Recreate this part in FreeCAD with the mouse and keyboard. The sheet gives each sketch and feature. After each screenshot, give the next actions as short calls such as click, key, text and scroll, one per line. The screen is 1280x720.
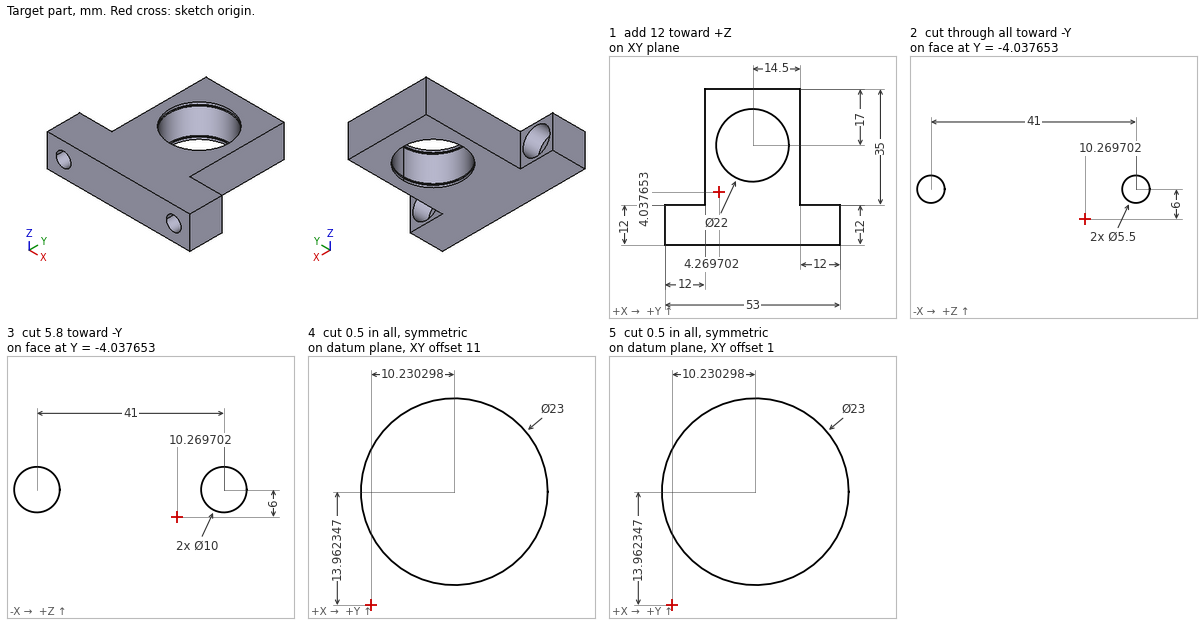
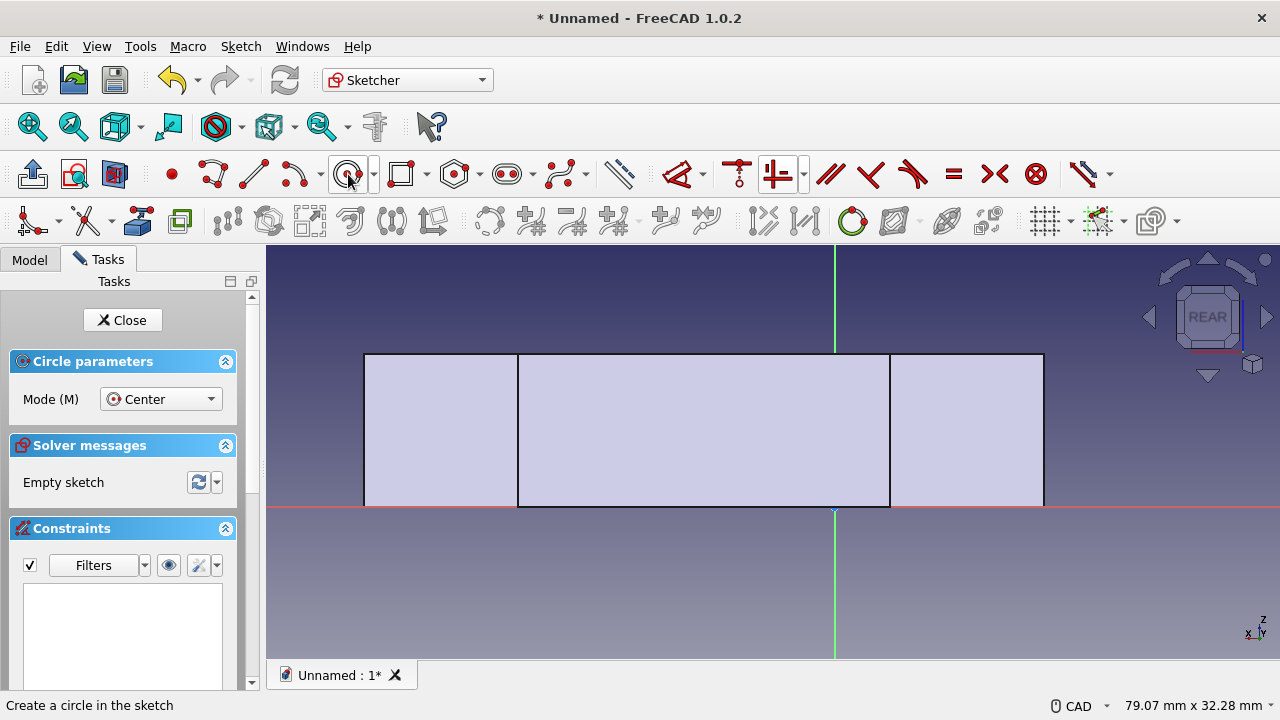
click(967, 431)
click(992, 406)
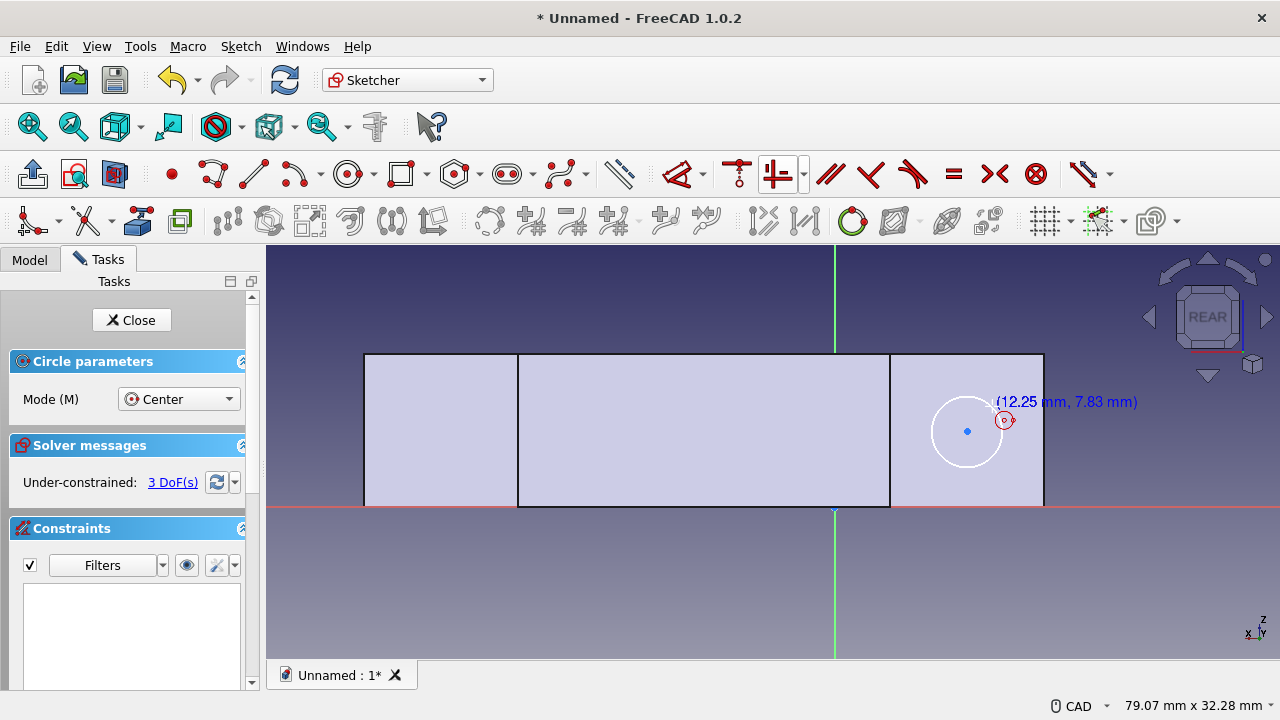
click(441, 431)
click(466, 406)
key(Escape)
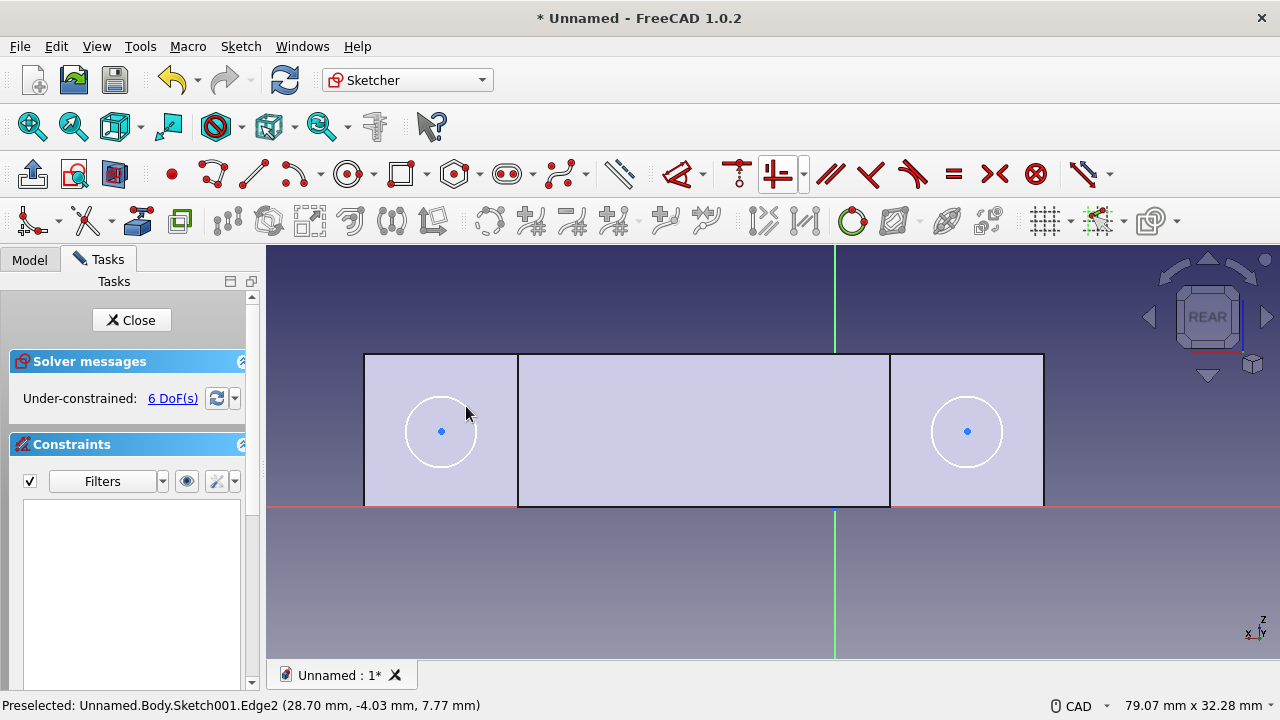
click(992, 407)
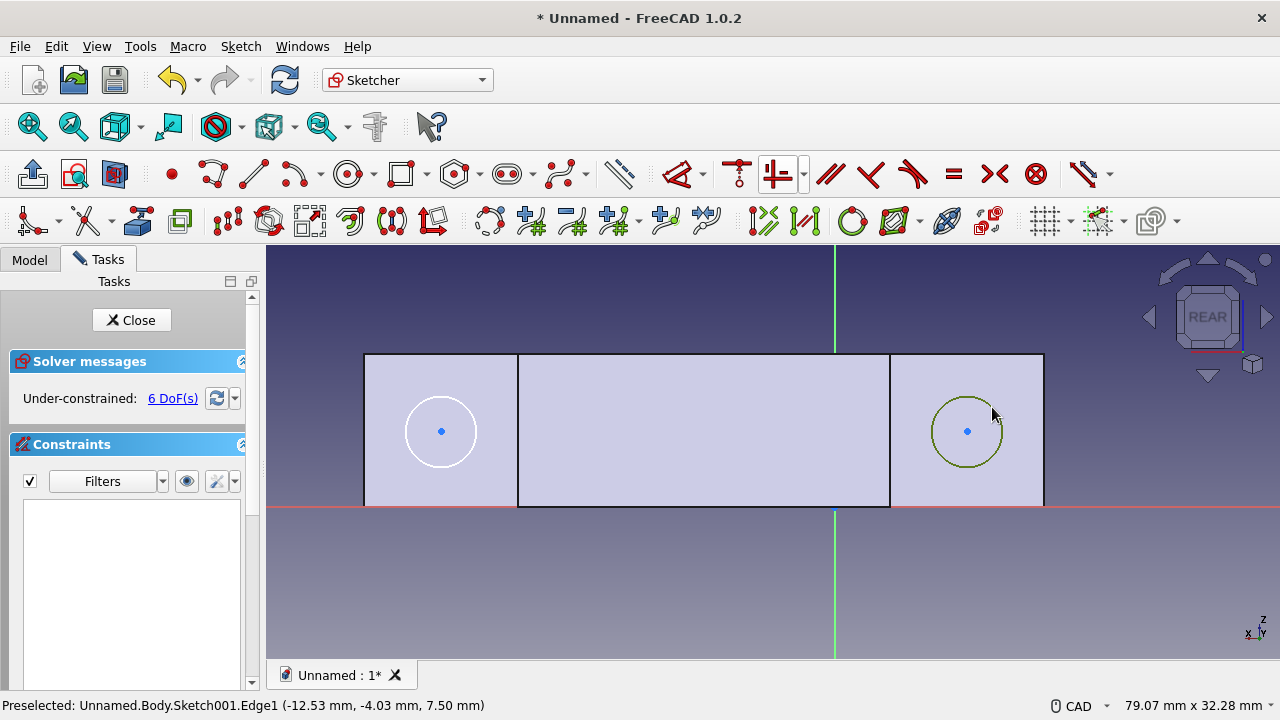
click(466, 407)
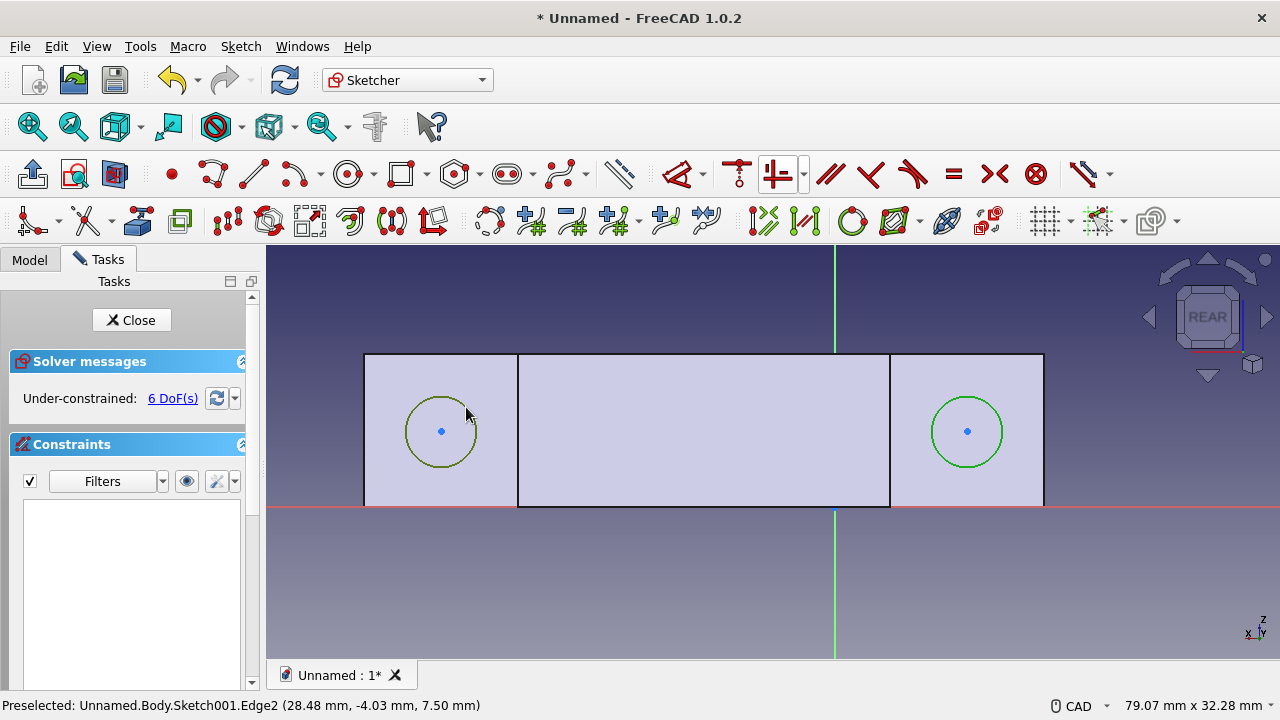
click(954, 174)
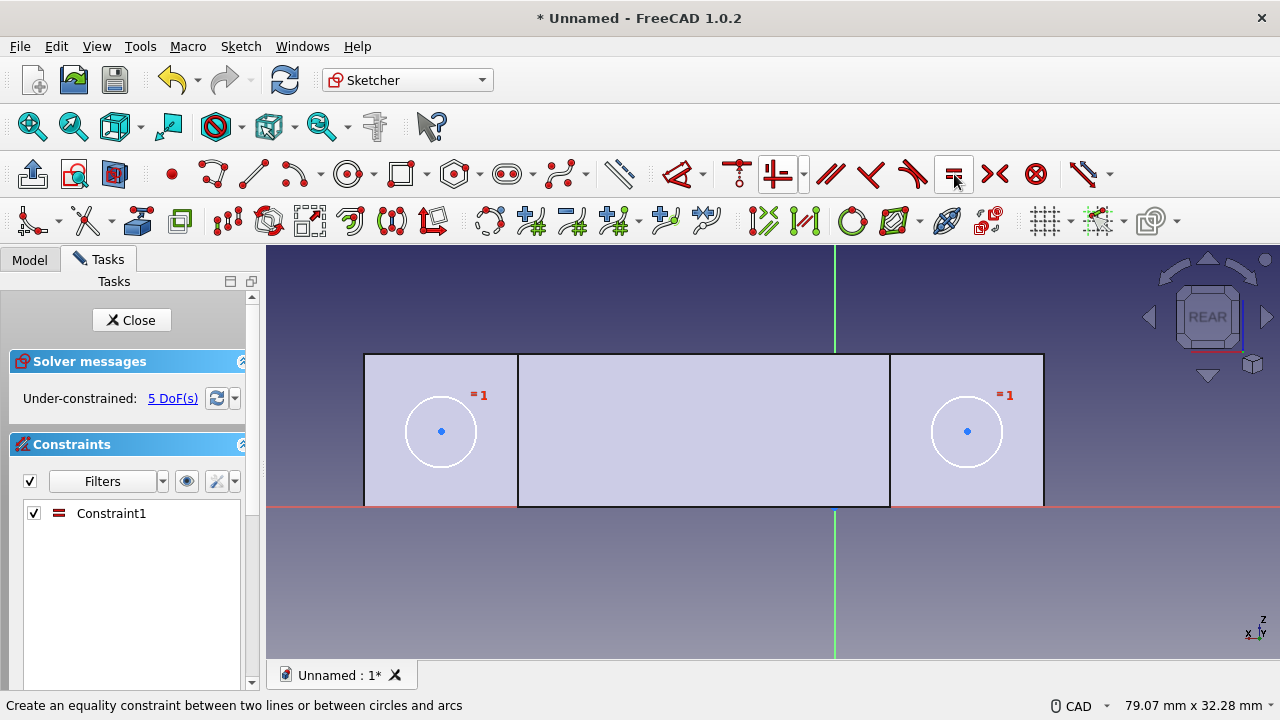
click(967, 432)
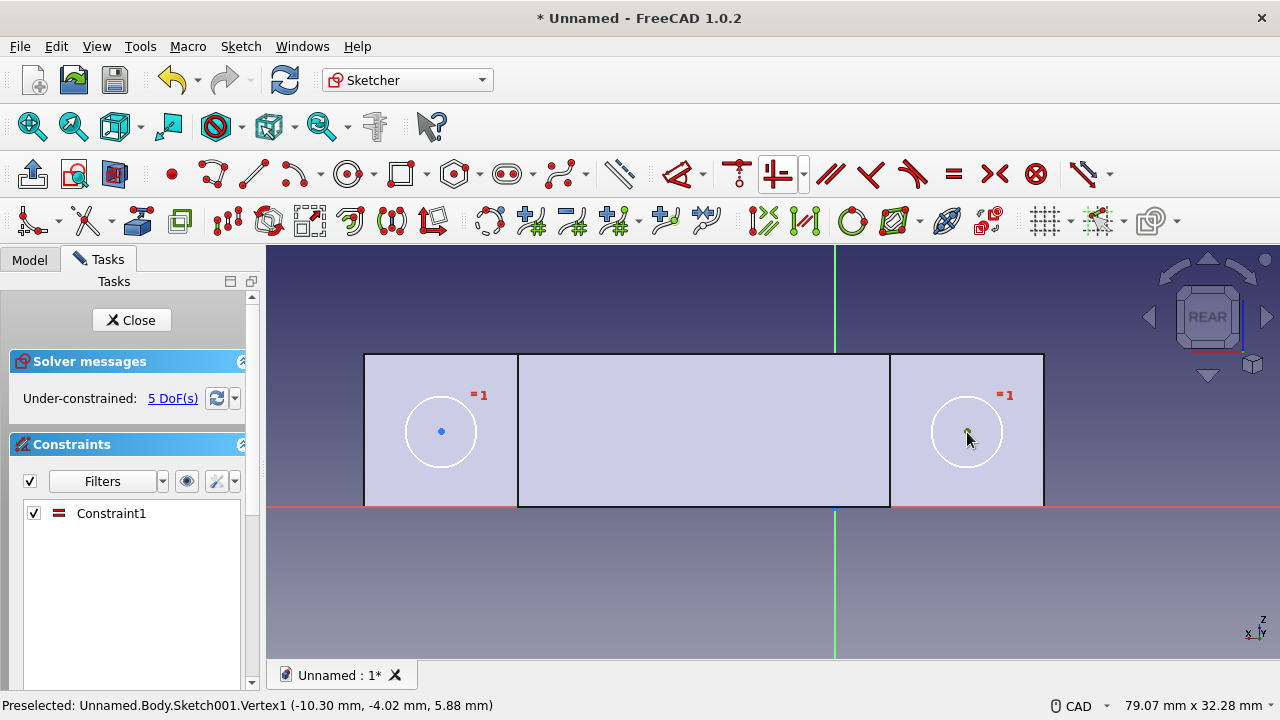
click(441, 432)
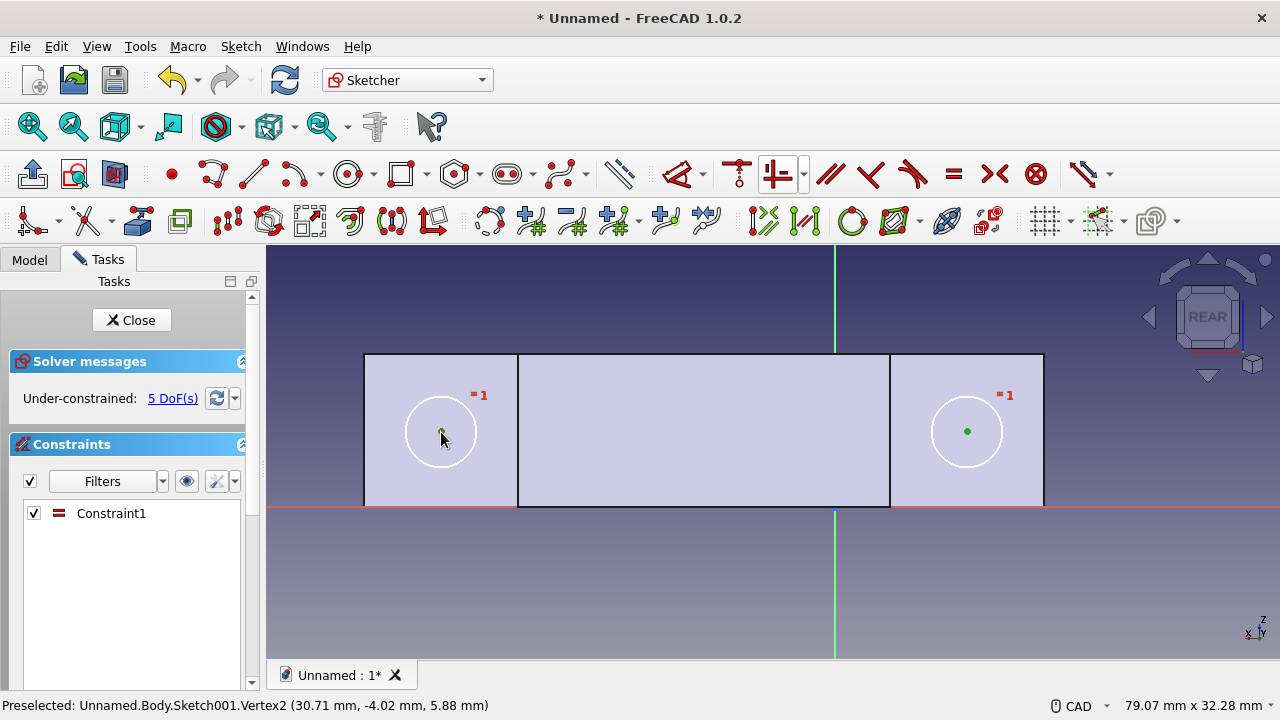
key(h)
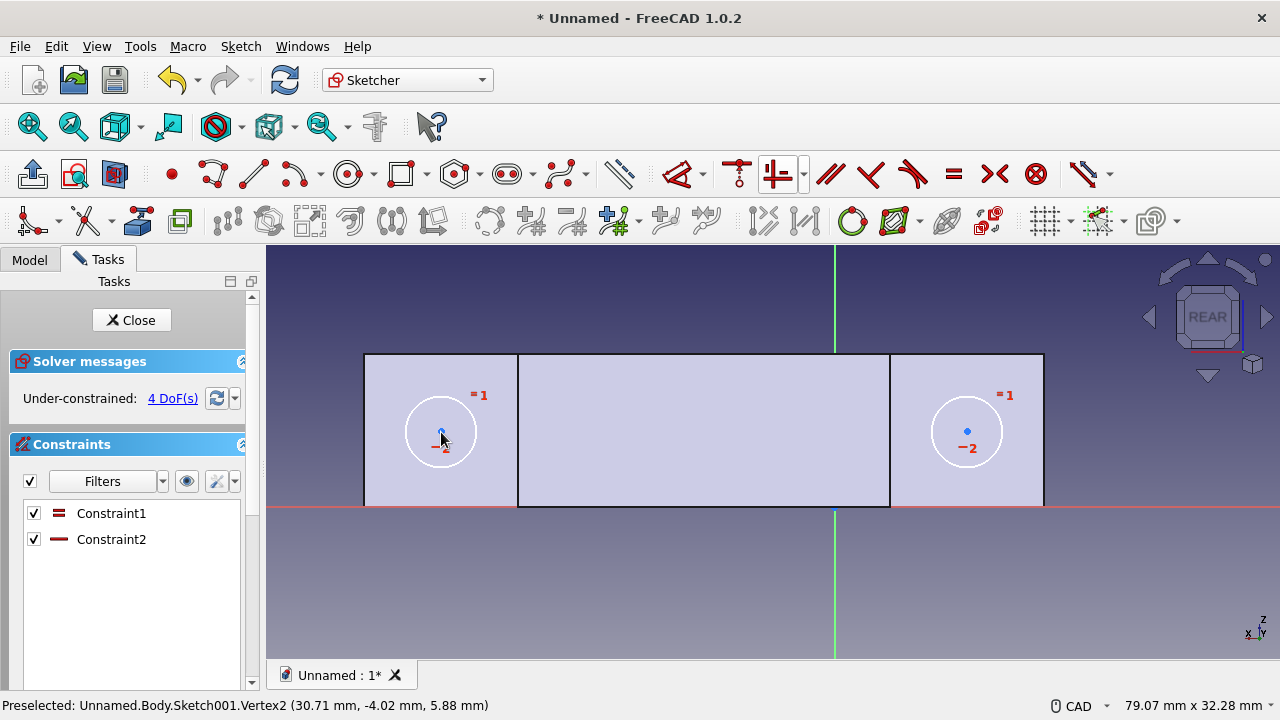
click(676, 174)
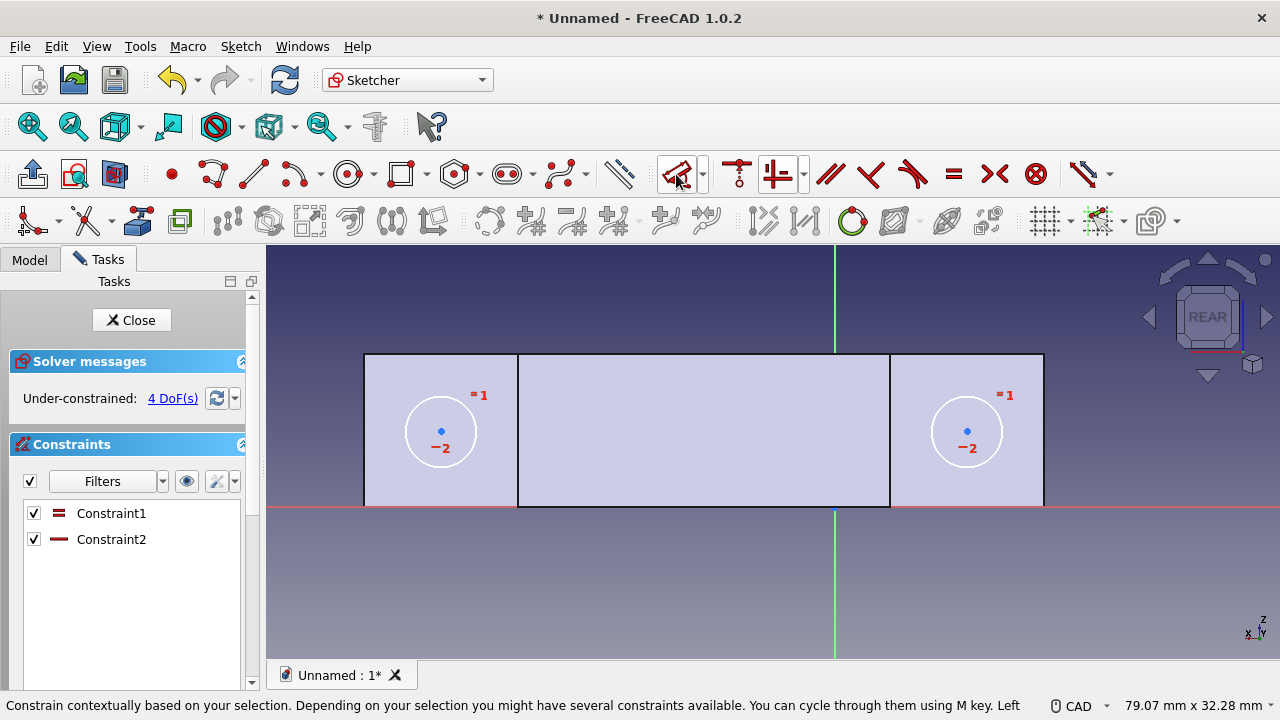
click(992, 407)
click(1015, 384)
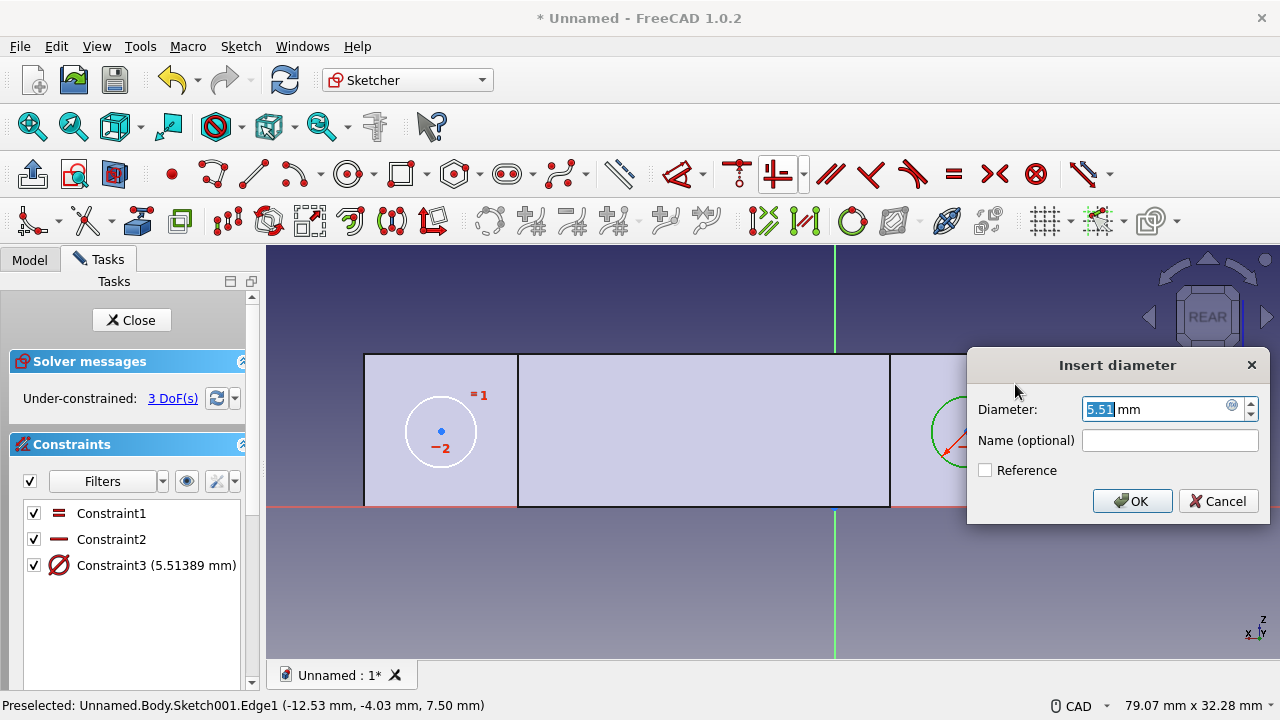
text(5.5)
key(Return)